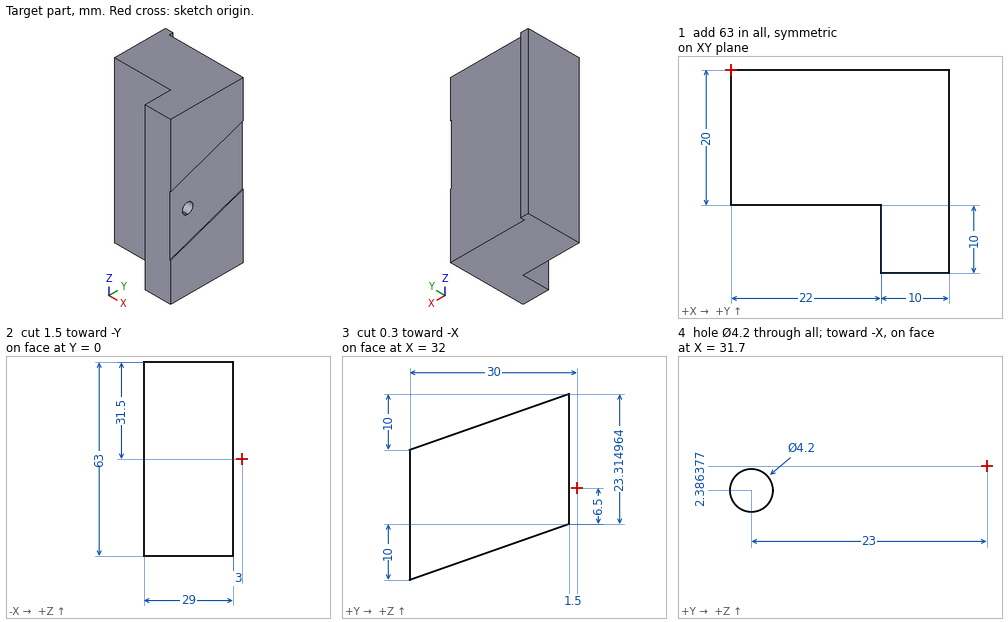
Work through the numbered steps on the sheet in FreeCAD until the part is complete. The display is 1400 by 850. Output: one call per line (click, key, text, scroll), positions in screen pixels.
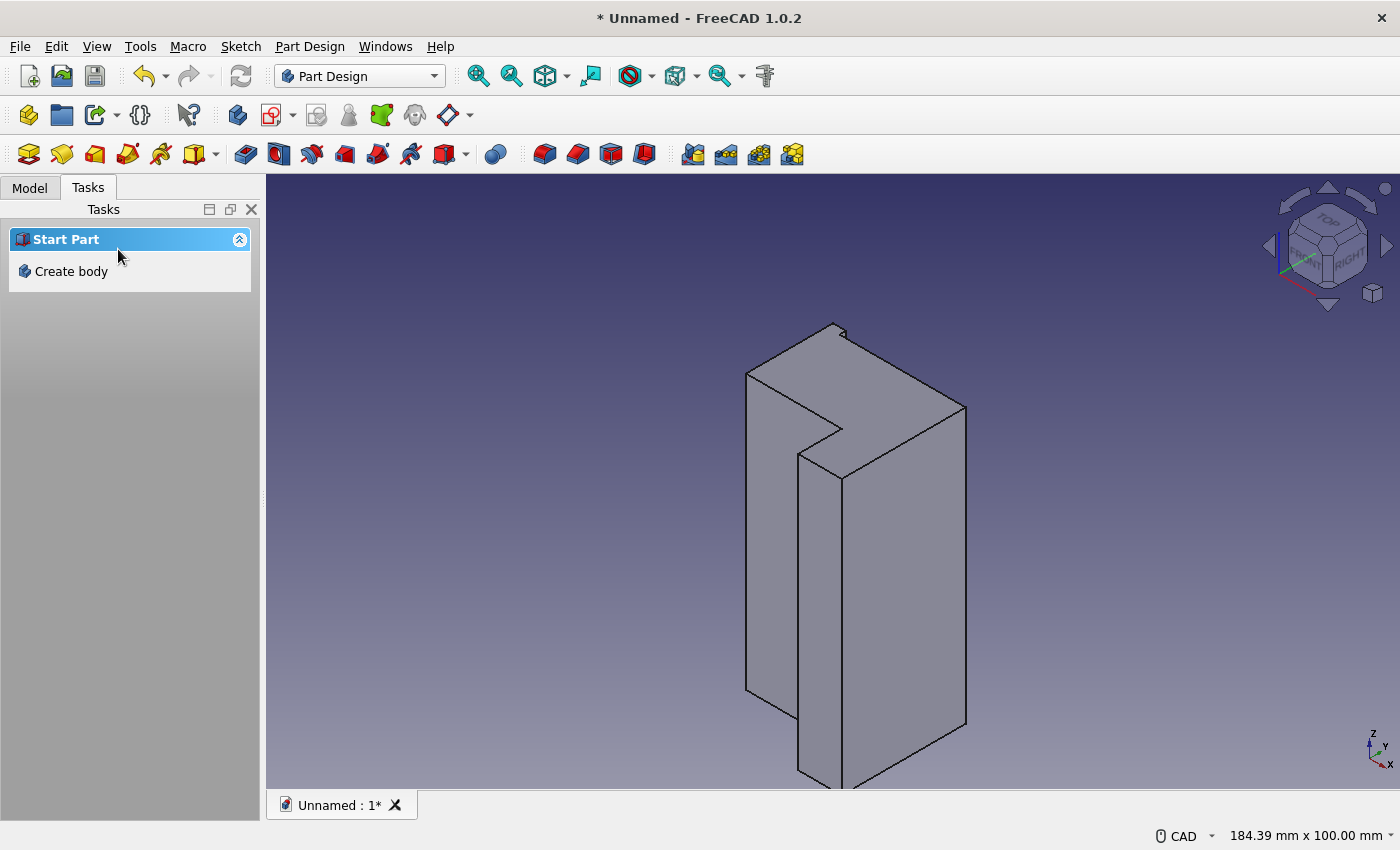
click(479, 76)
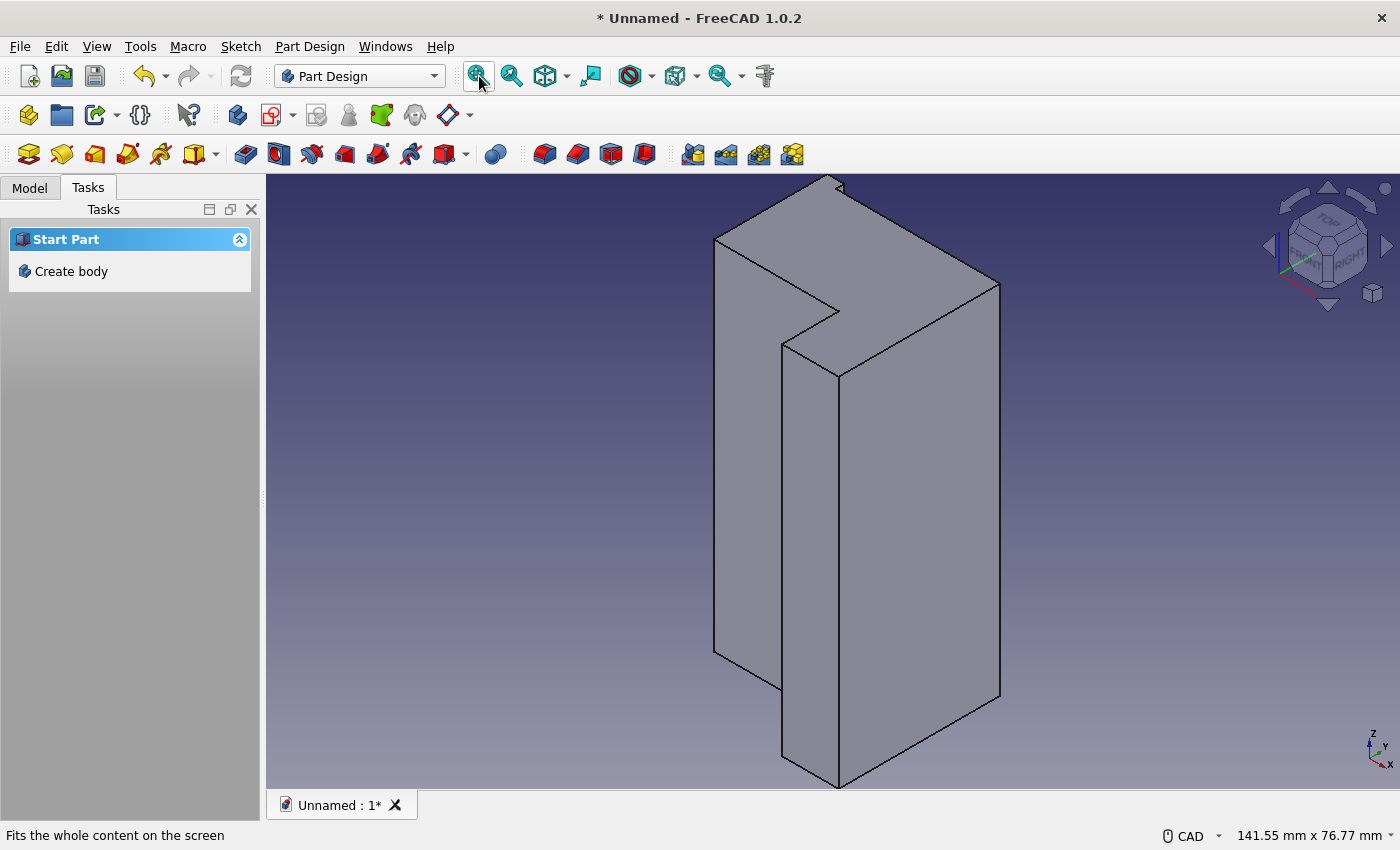
click(919, 476)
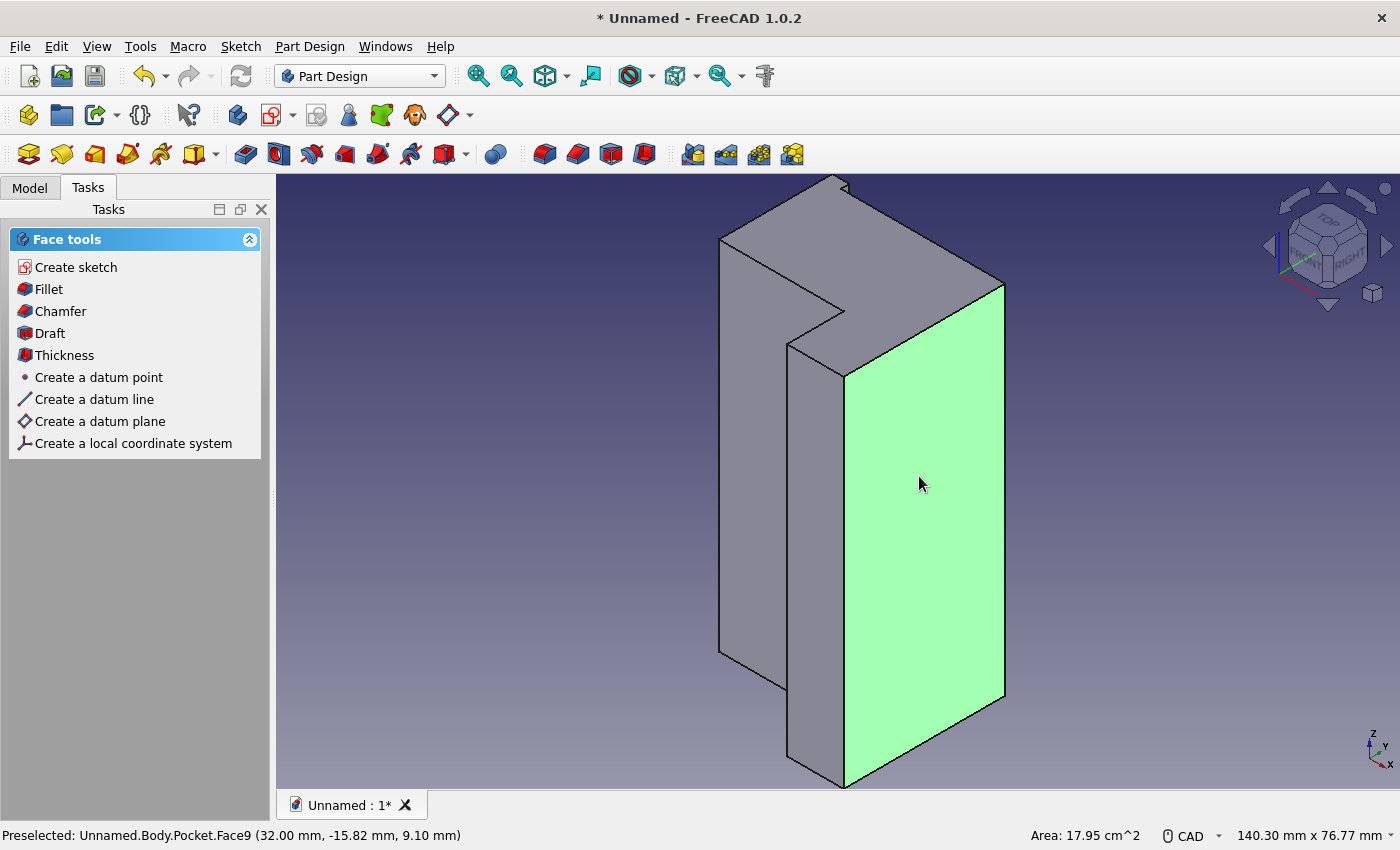
click(270, 116)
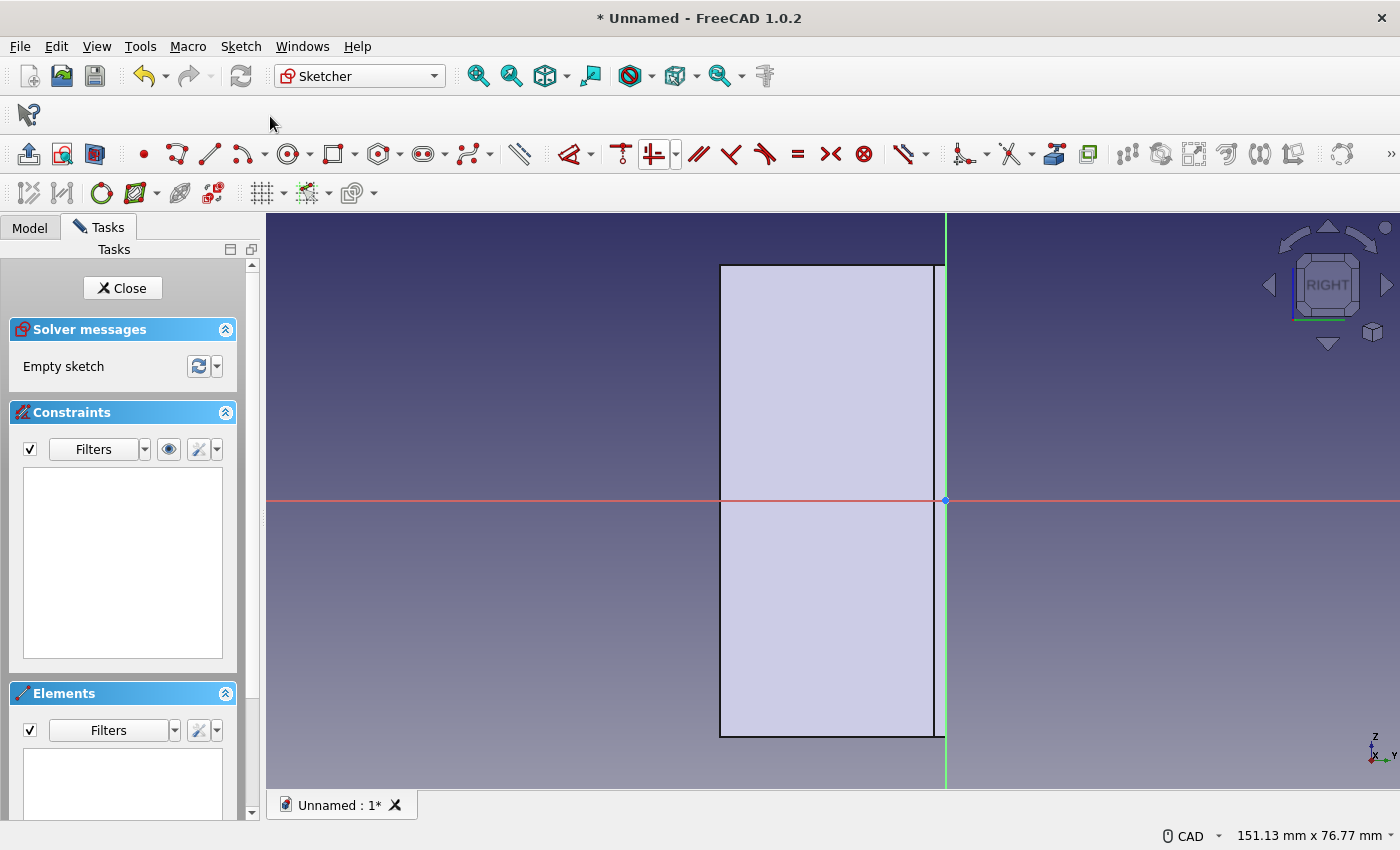
scroll(972, 497, up, 2)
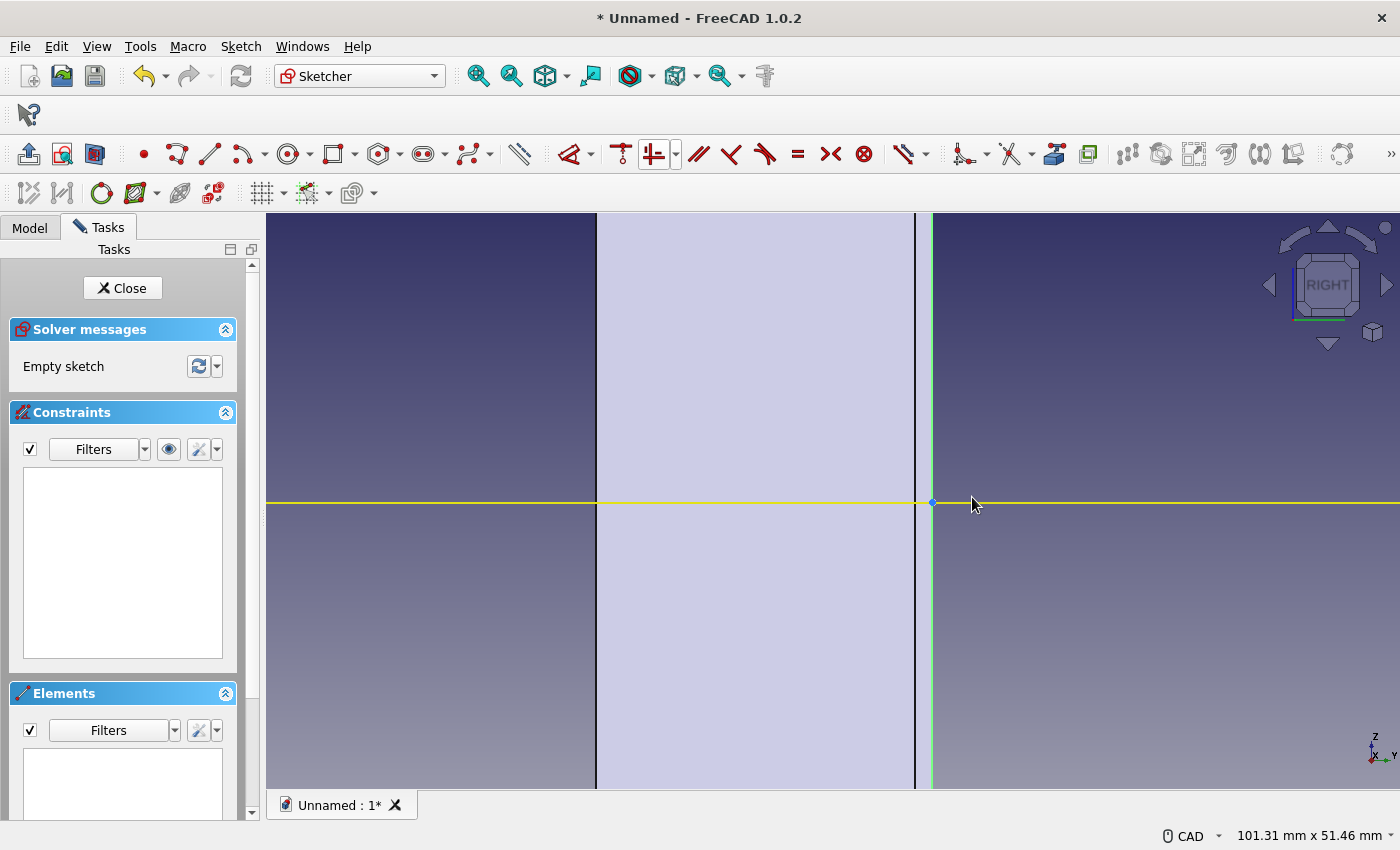
click(177, 154)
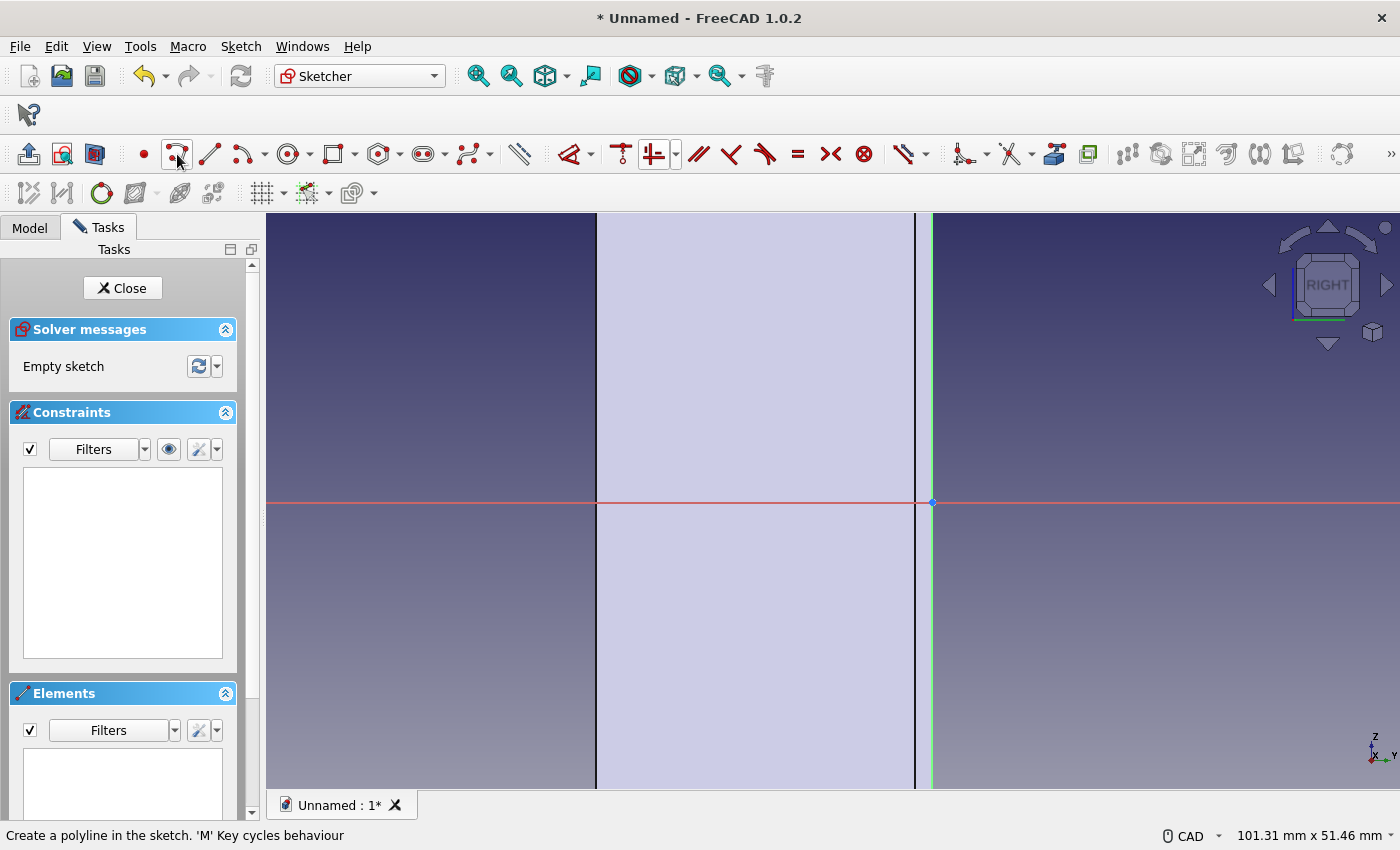
click(915, 575)
click(915, 315)
click(596, 426)
click(596, 687)
click(915, 576)
key(Escape)
key(Escape)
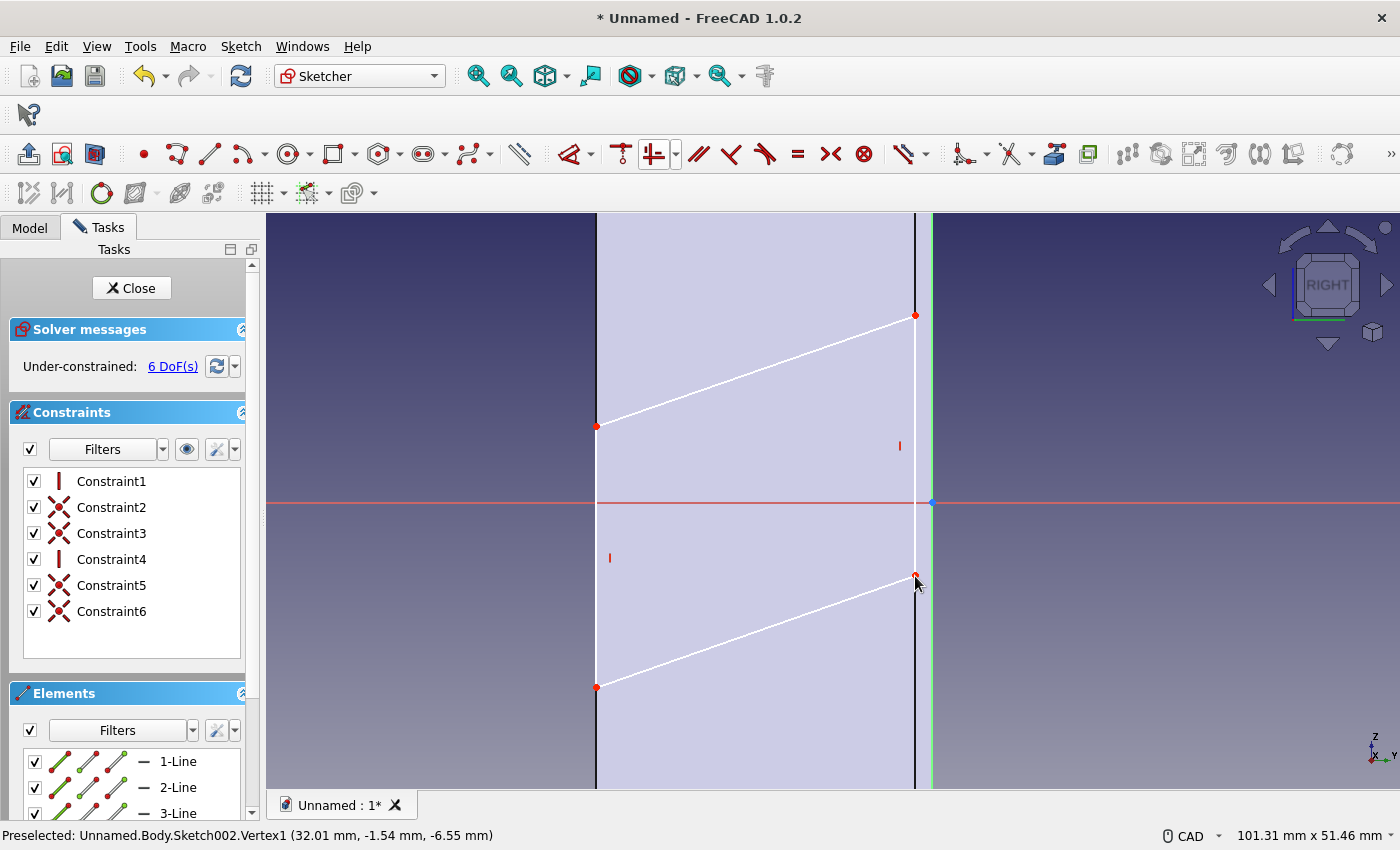
click(568, 154)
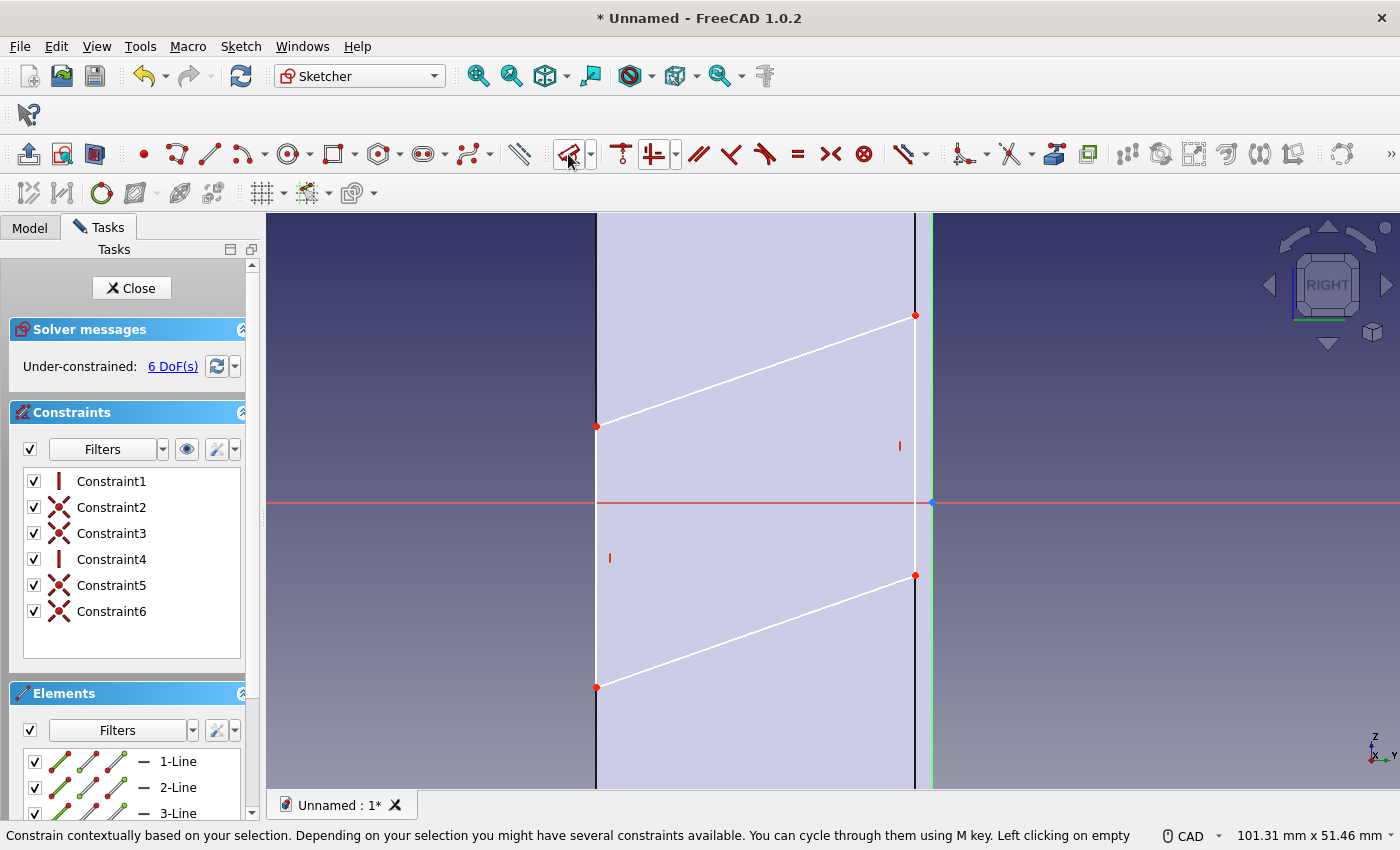
click(596, 427)
click(764, 393)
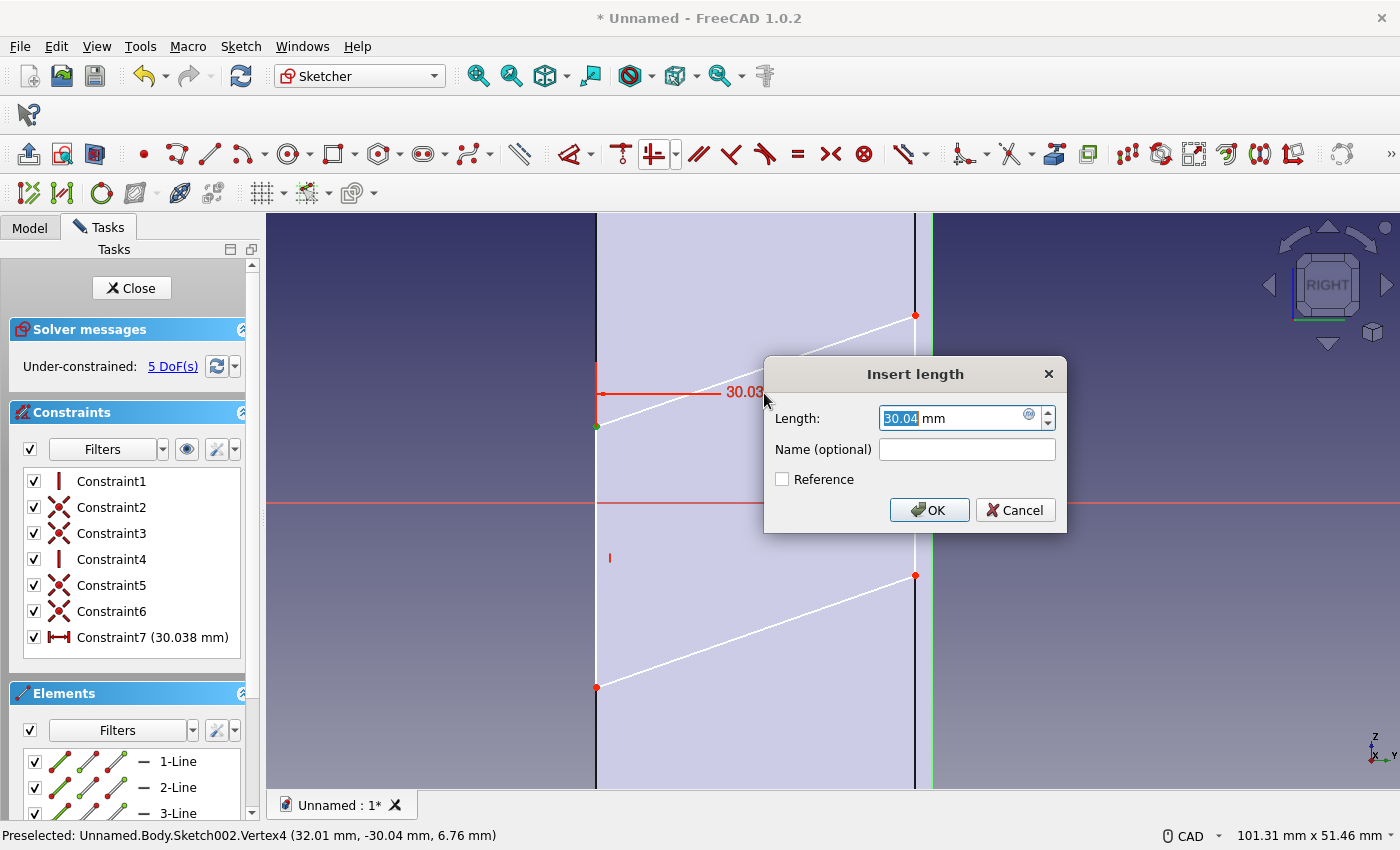
text(30)
key(Return)